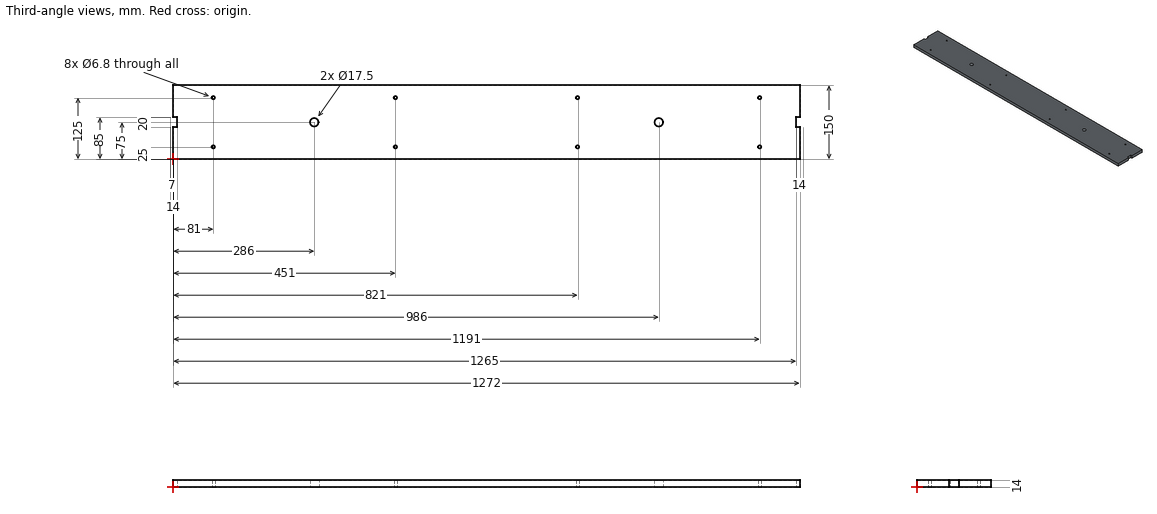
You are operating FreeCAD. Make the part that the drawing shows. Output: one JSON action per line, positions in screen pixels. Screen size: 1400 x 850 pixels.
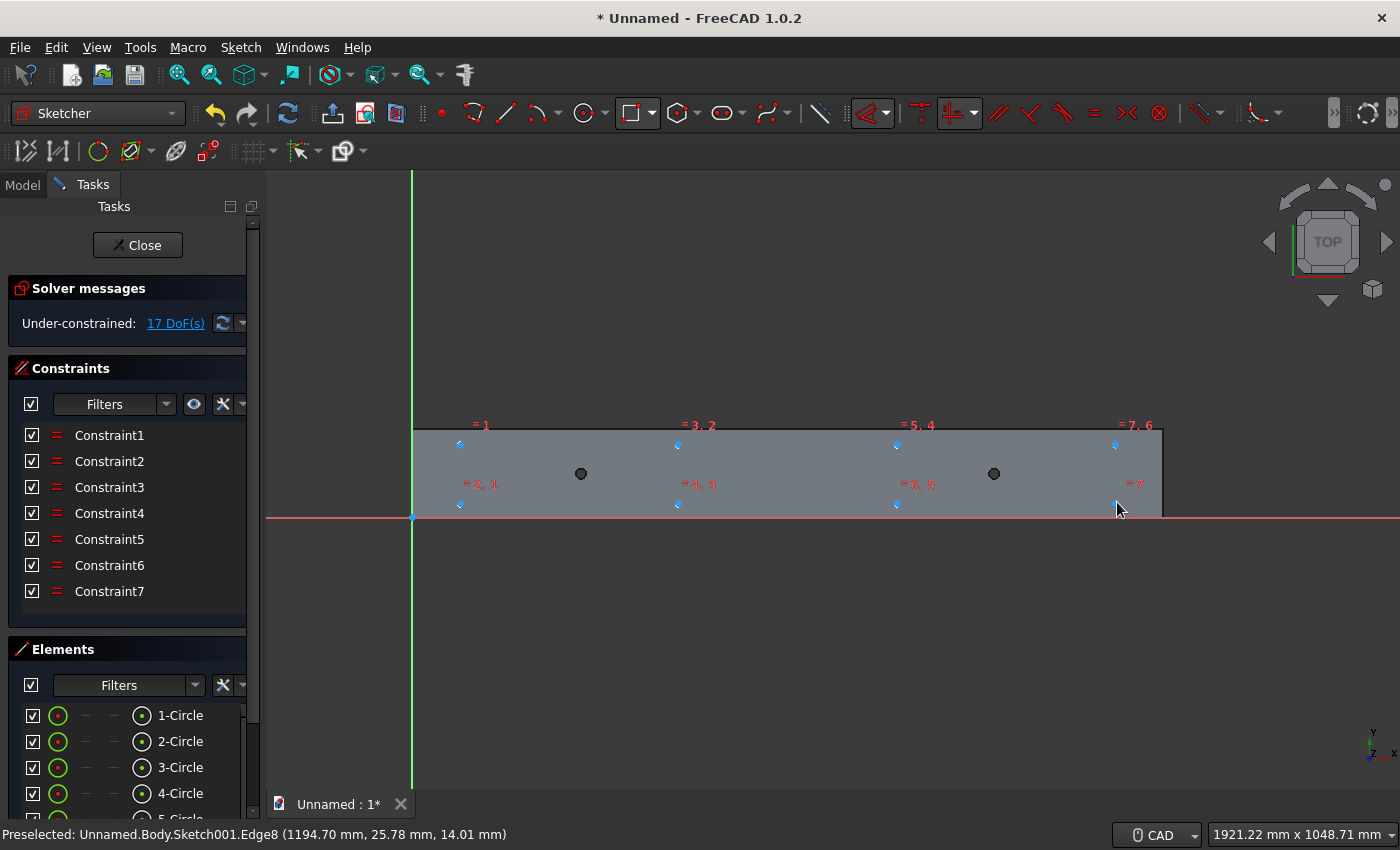
{"action": "left_click", "coordinate": [460, 445]}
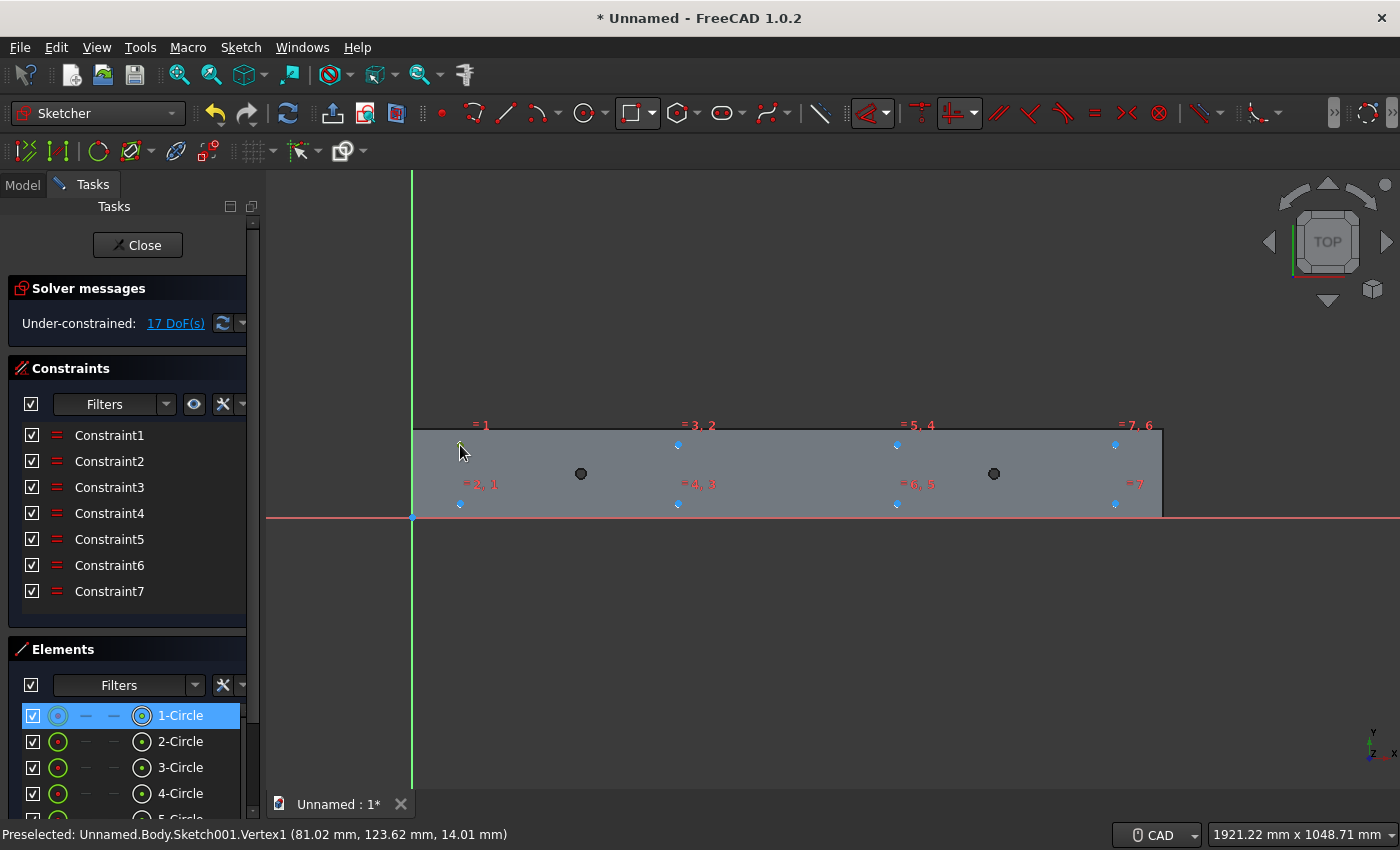
{"action": "left_click", "coordinate": [460, 504]}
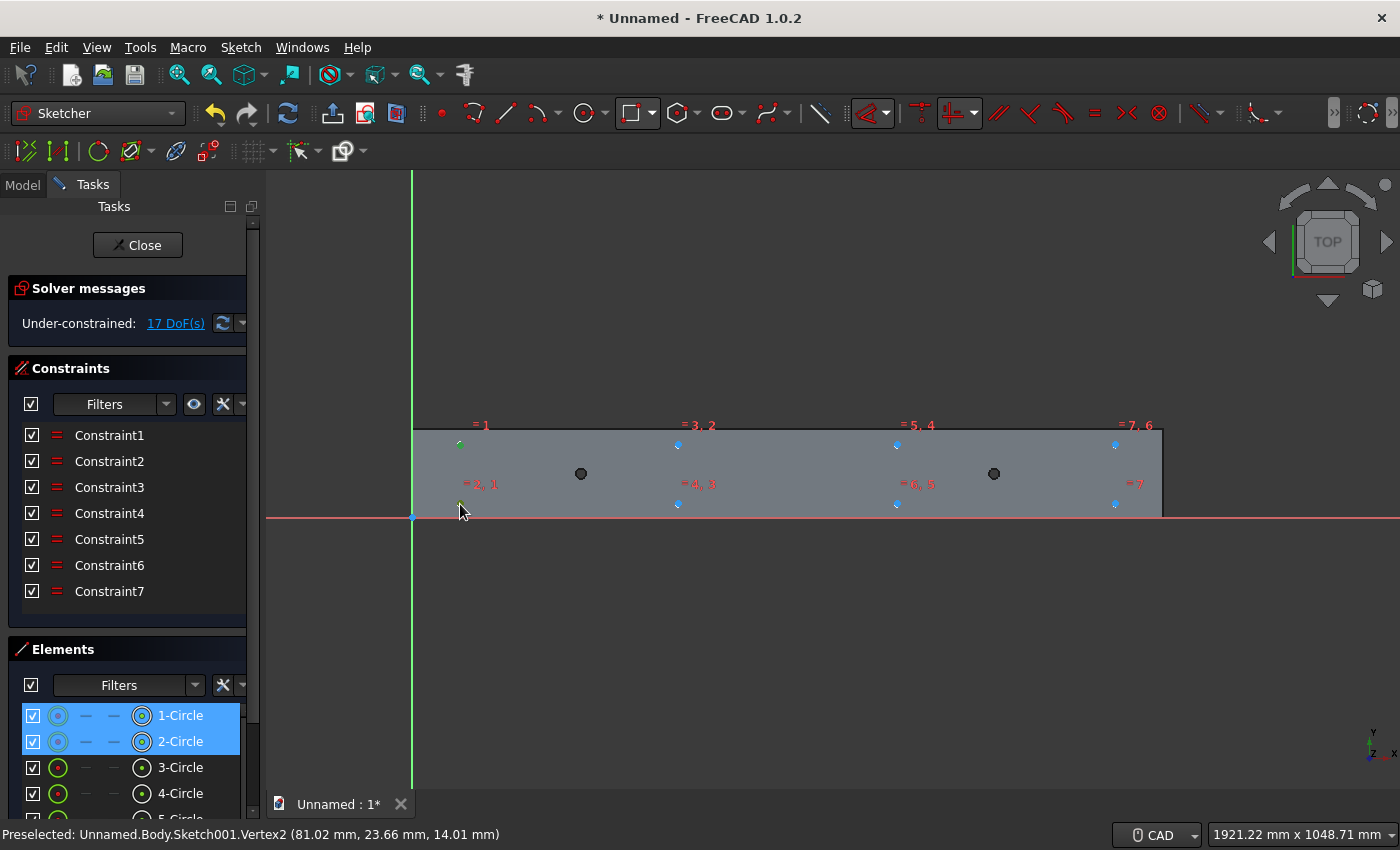
{"action": "key", "text": "v"}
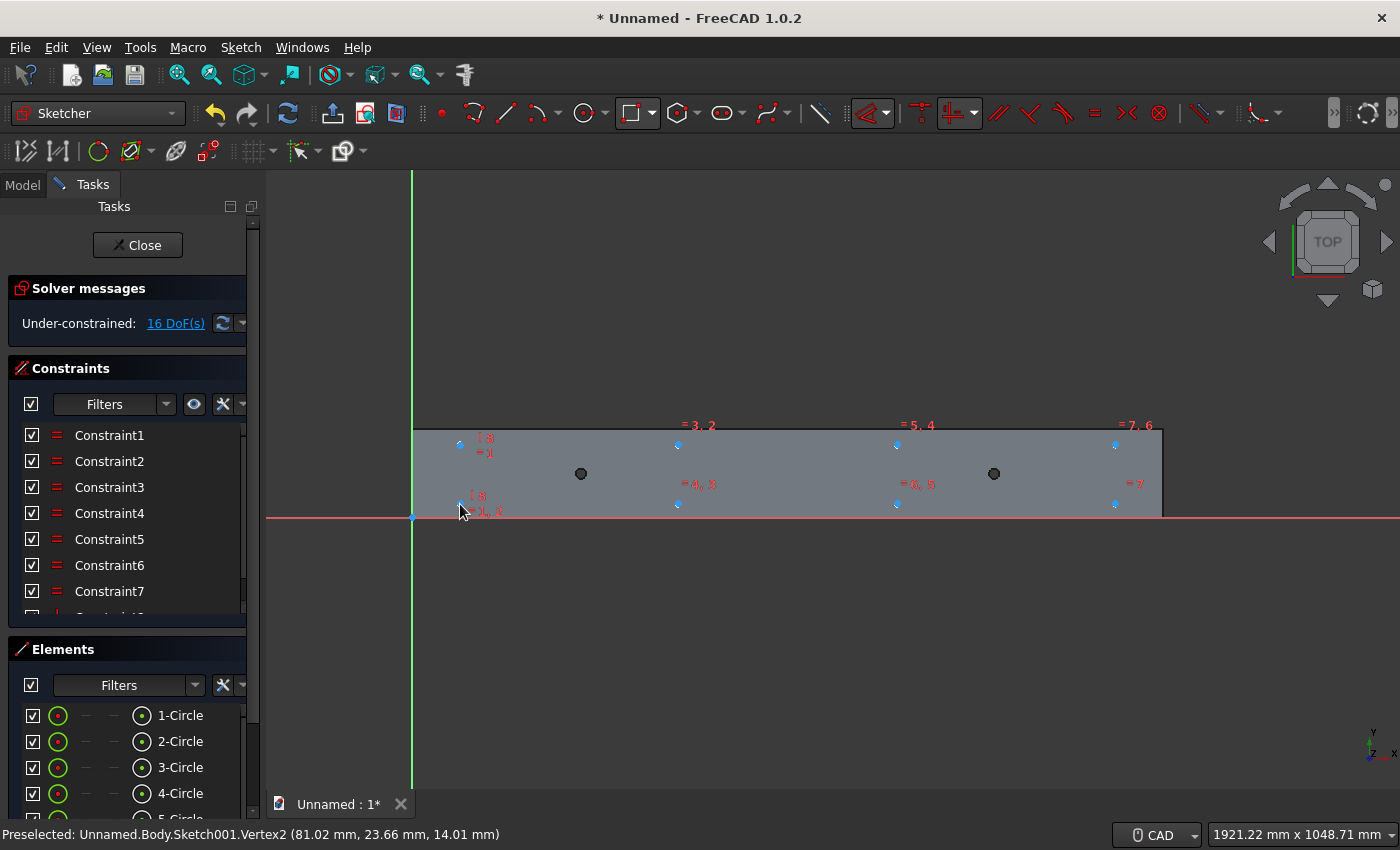
{"action": "left_click", "coordinate": [460, 445]}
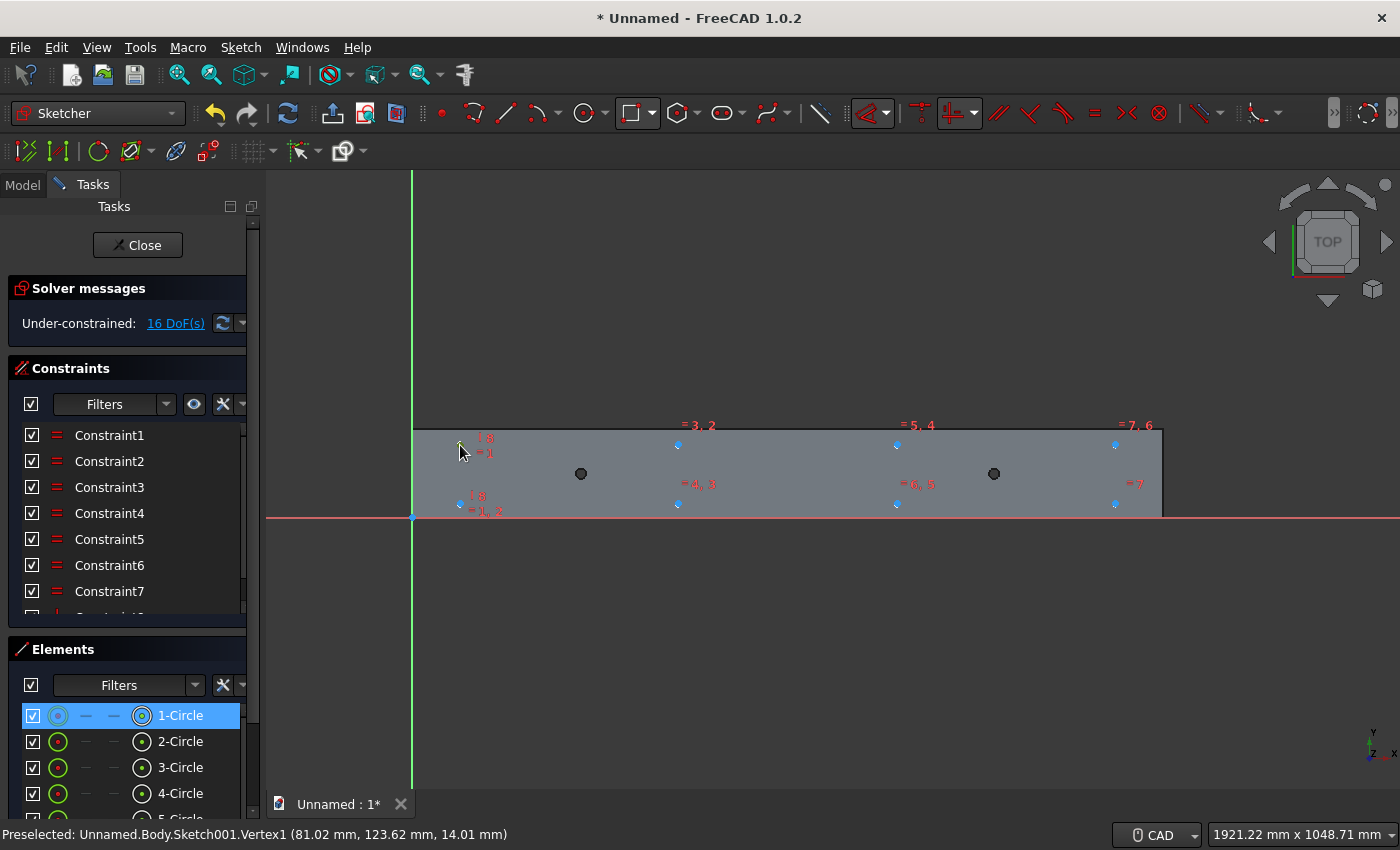
{"action": "left_click", "coordinate": [678, 445]}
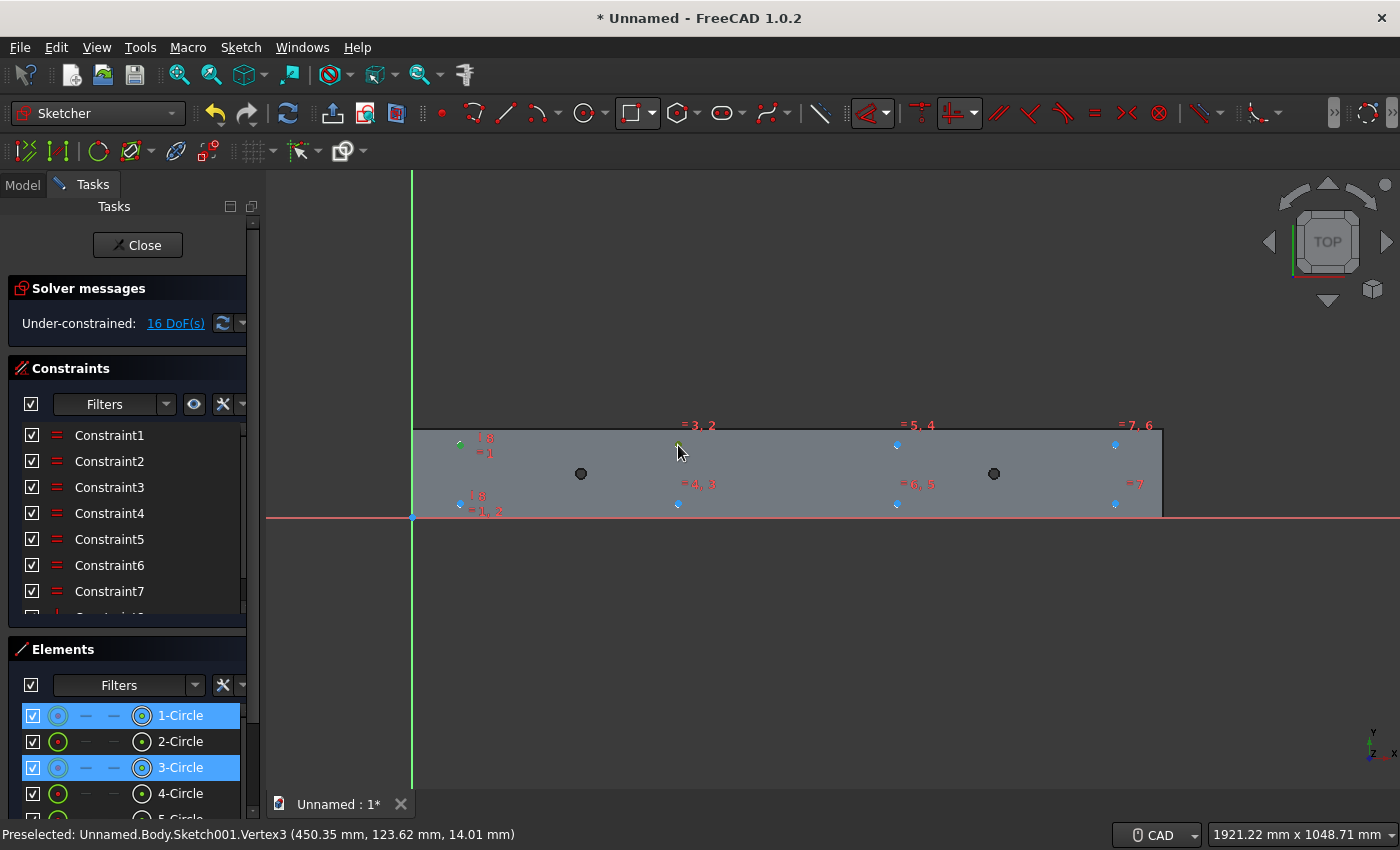
{"action": "left_click", "coordinate": [976, 114]}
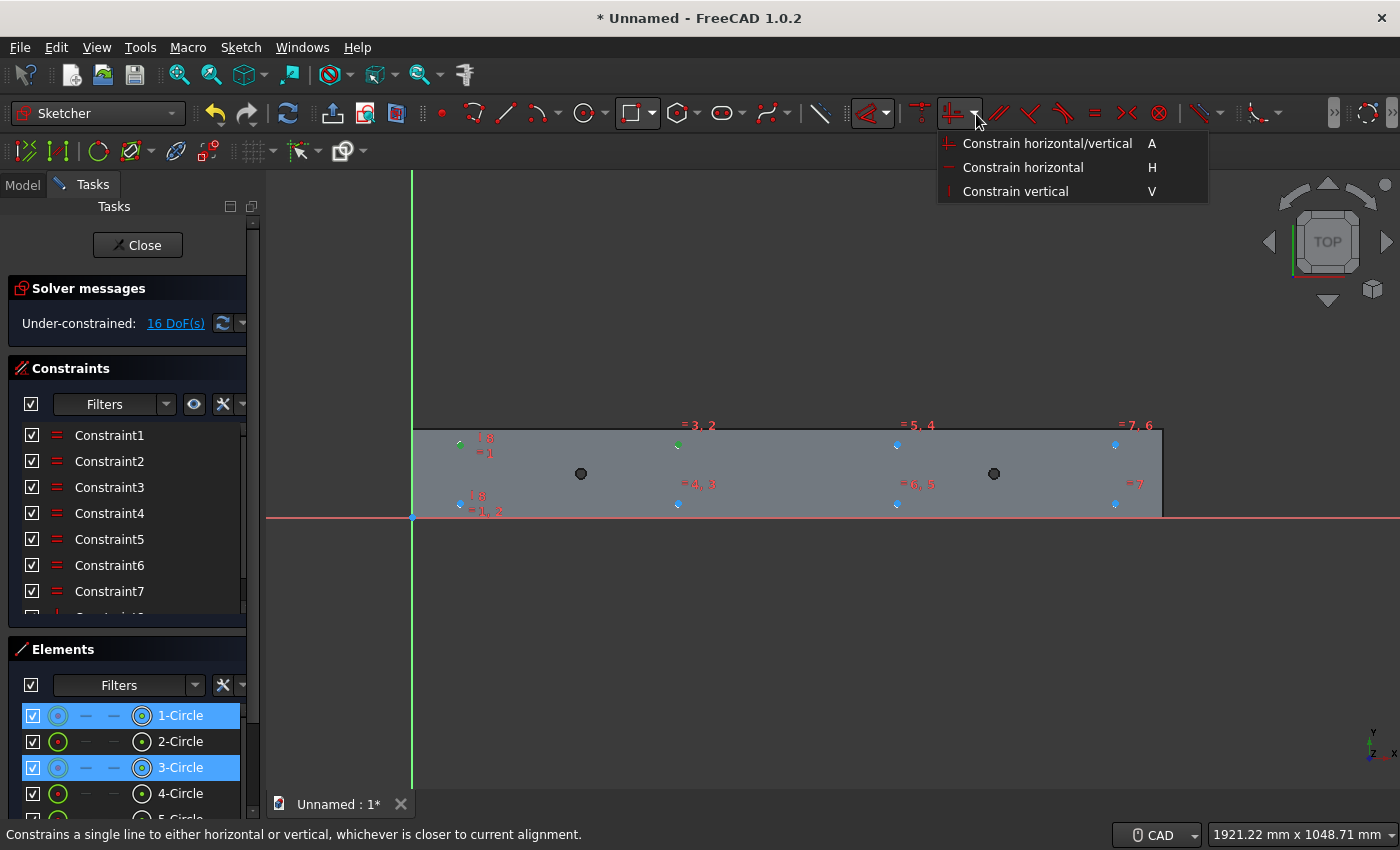
{"action": "left_click", "coordinate": [1073, 167]}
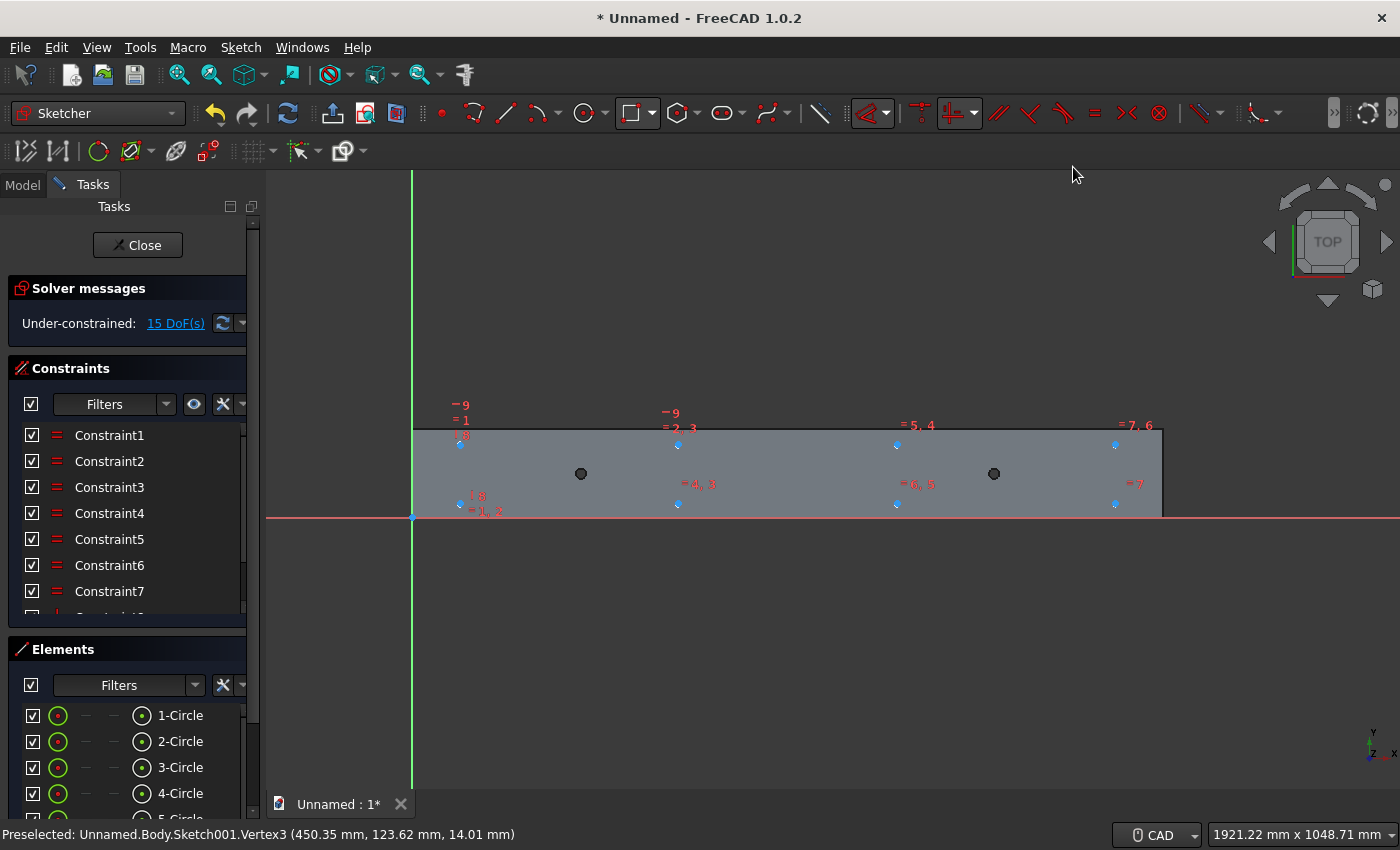
{"action": "left_click", "coordinate": [678, 445]}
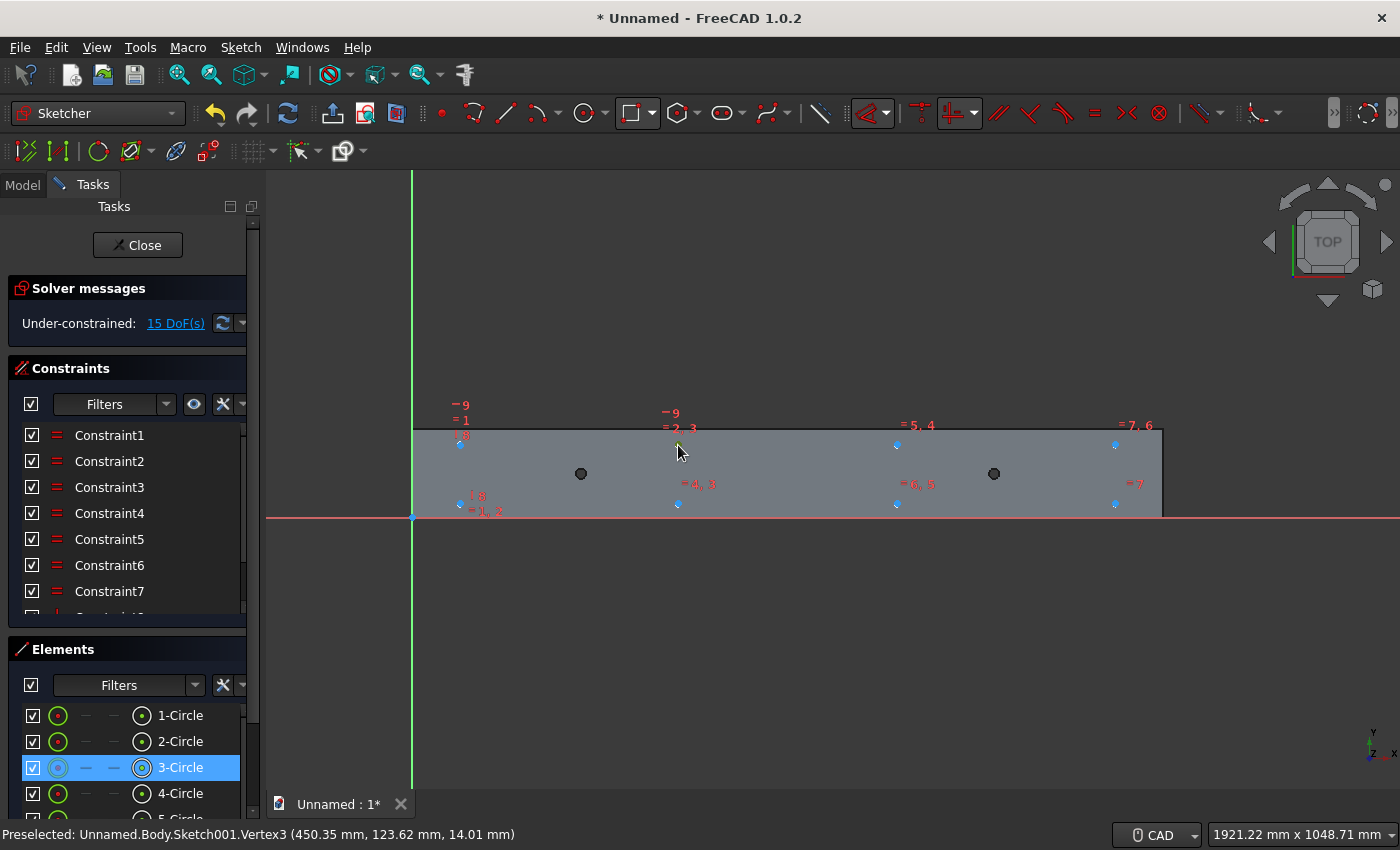
{"action": "left_click", "coordinate": [678, 504]}